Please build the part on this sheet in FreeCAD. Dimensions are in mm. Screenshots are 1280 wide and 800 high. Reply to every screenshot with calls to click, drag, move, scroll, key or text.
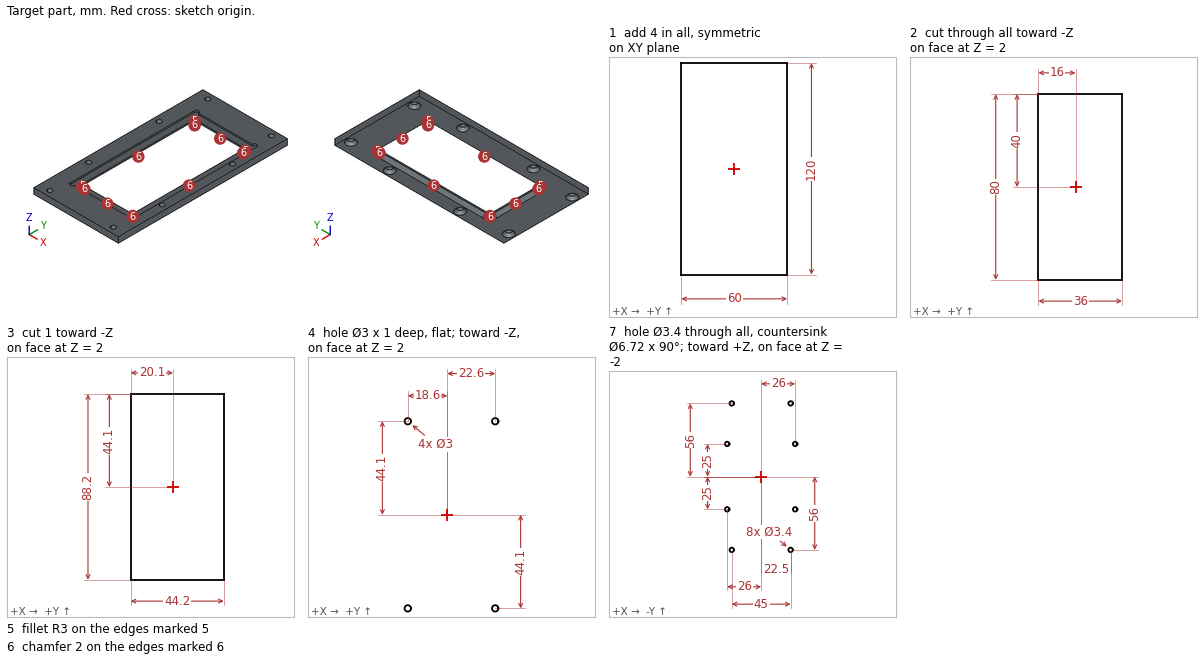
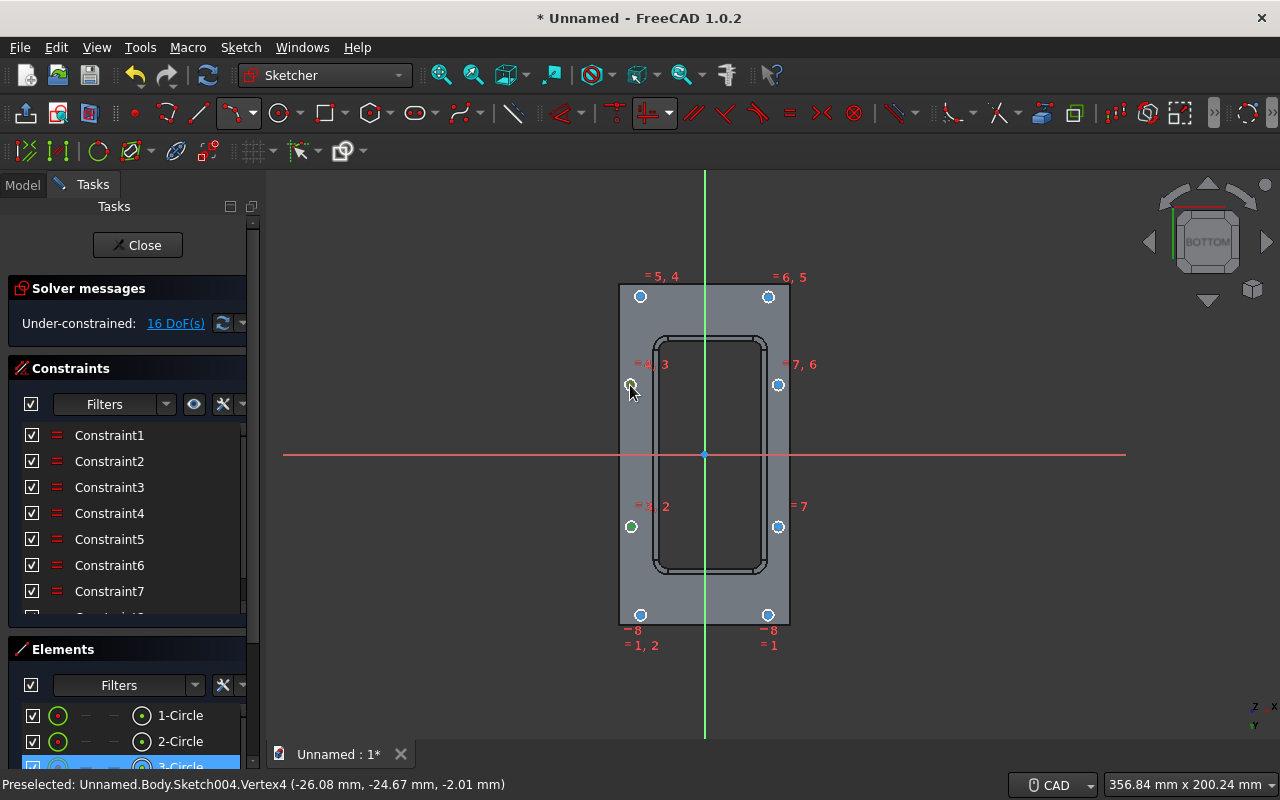
key(v)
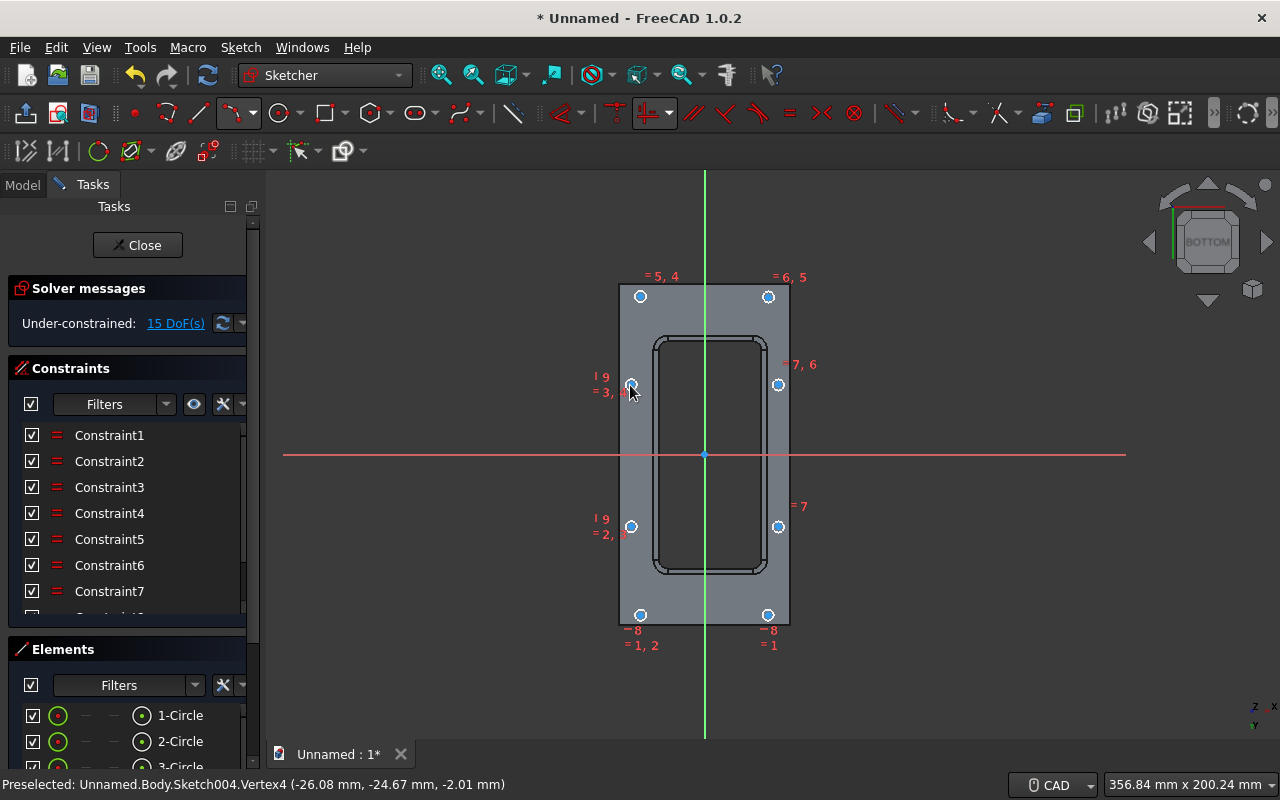
click(641, 615)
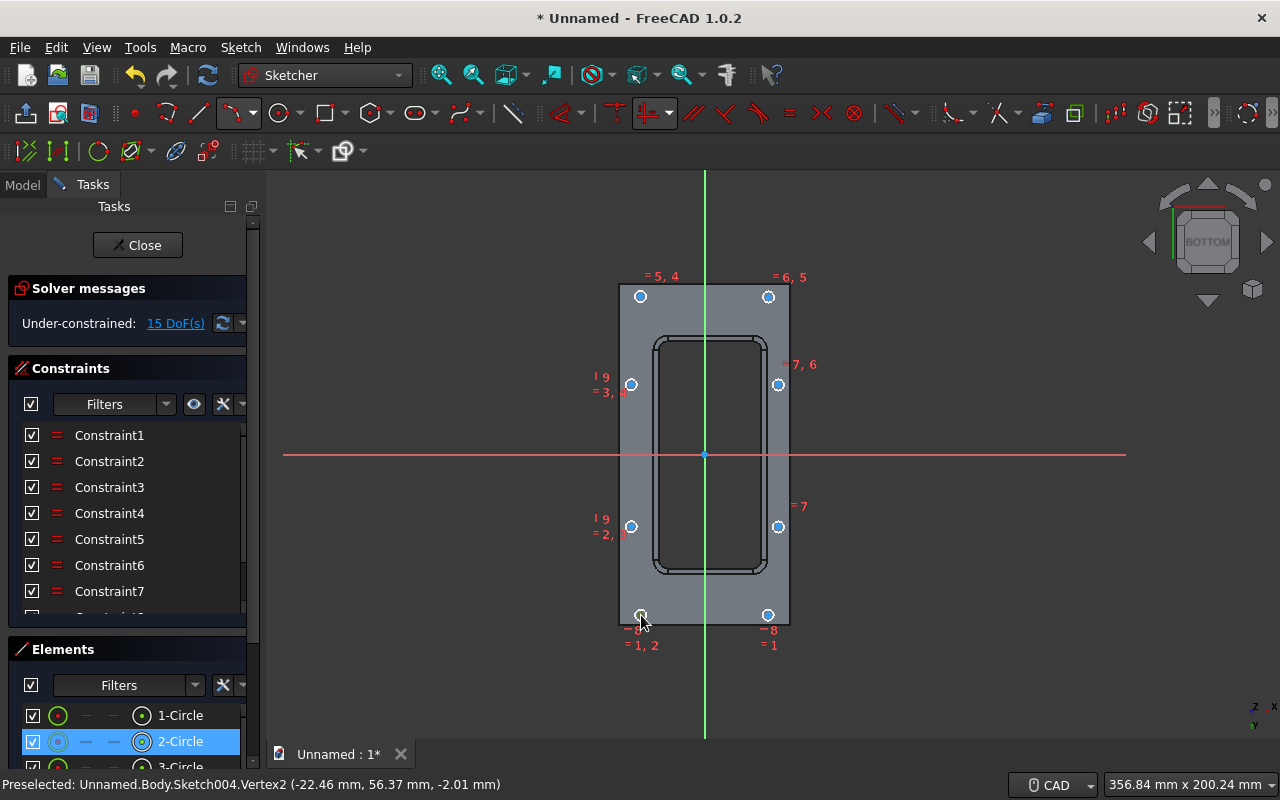
click(640, 297)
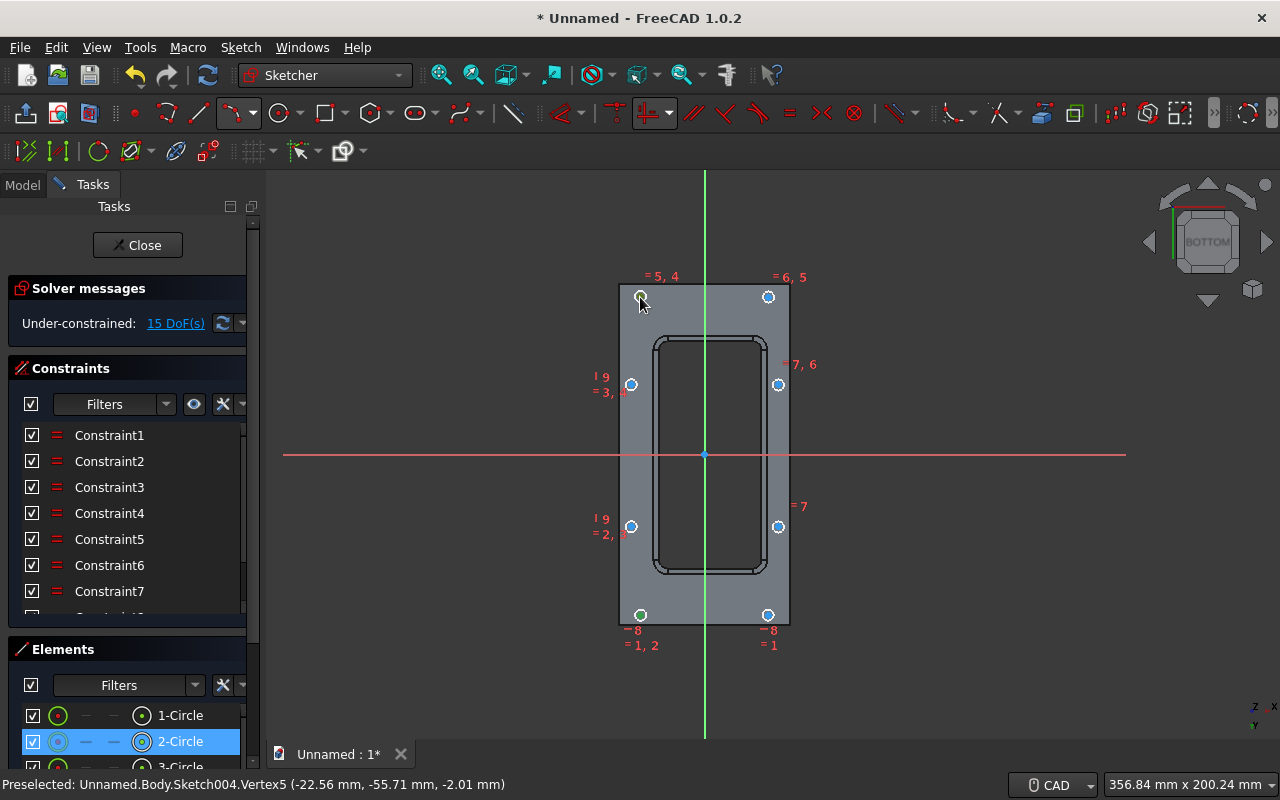
click(672, 114)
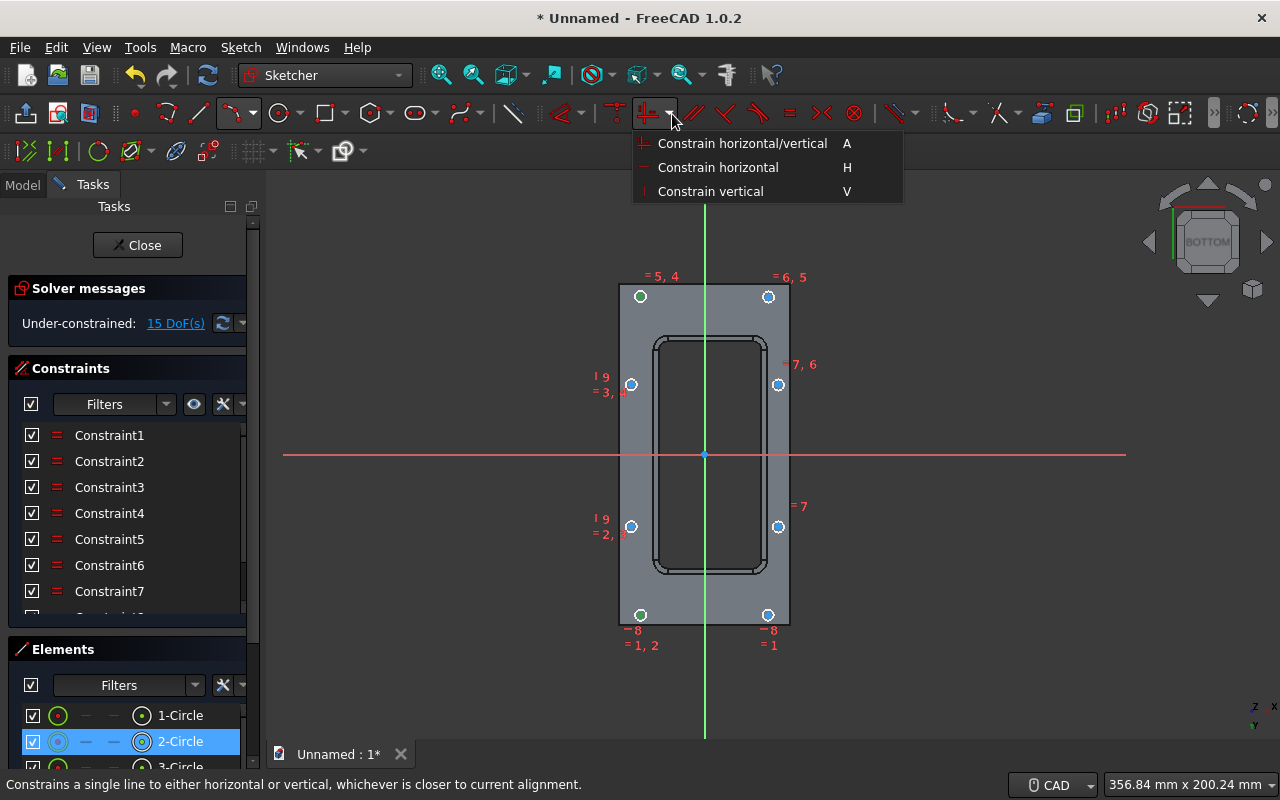
click(768, 191)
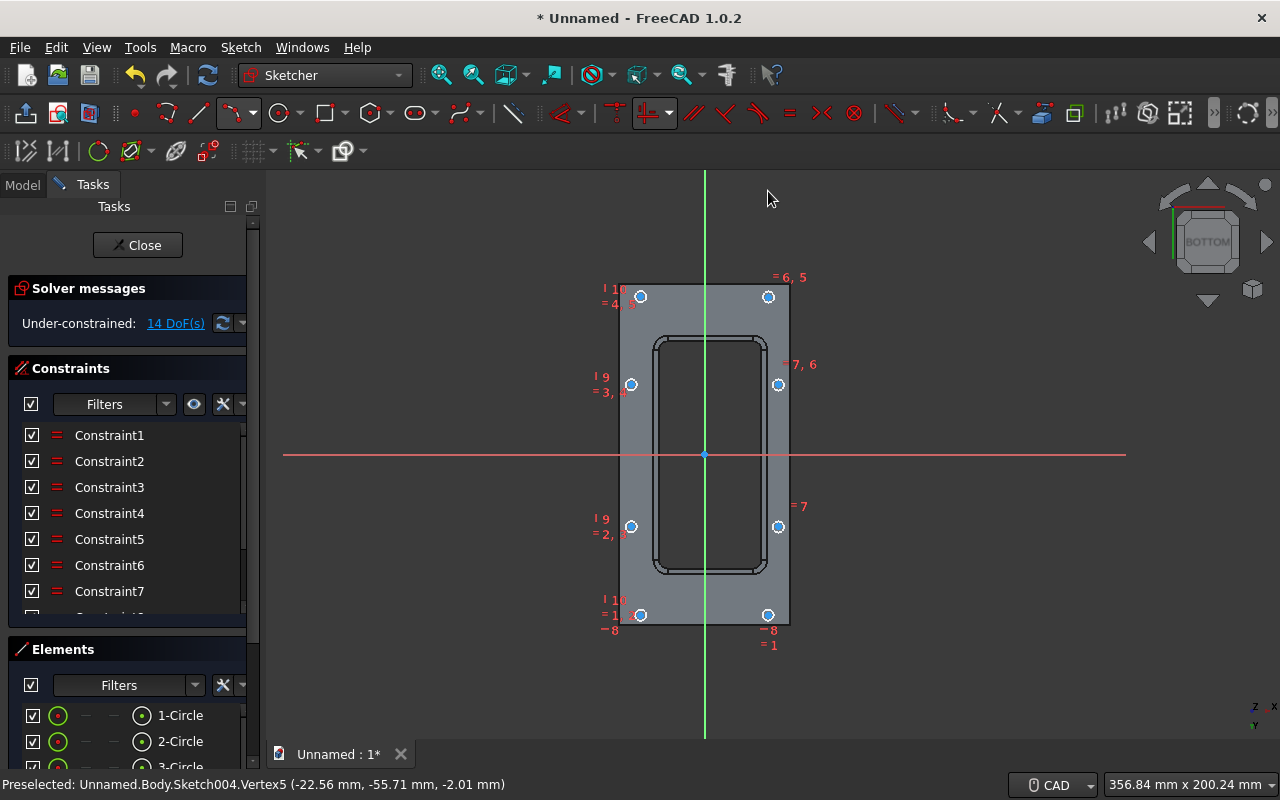
click(768, 615)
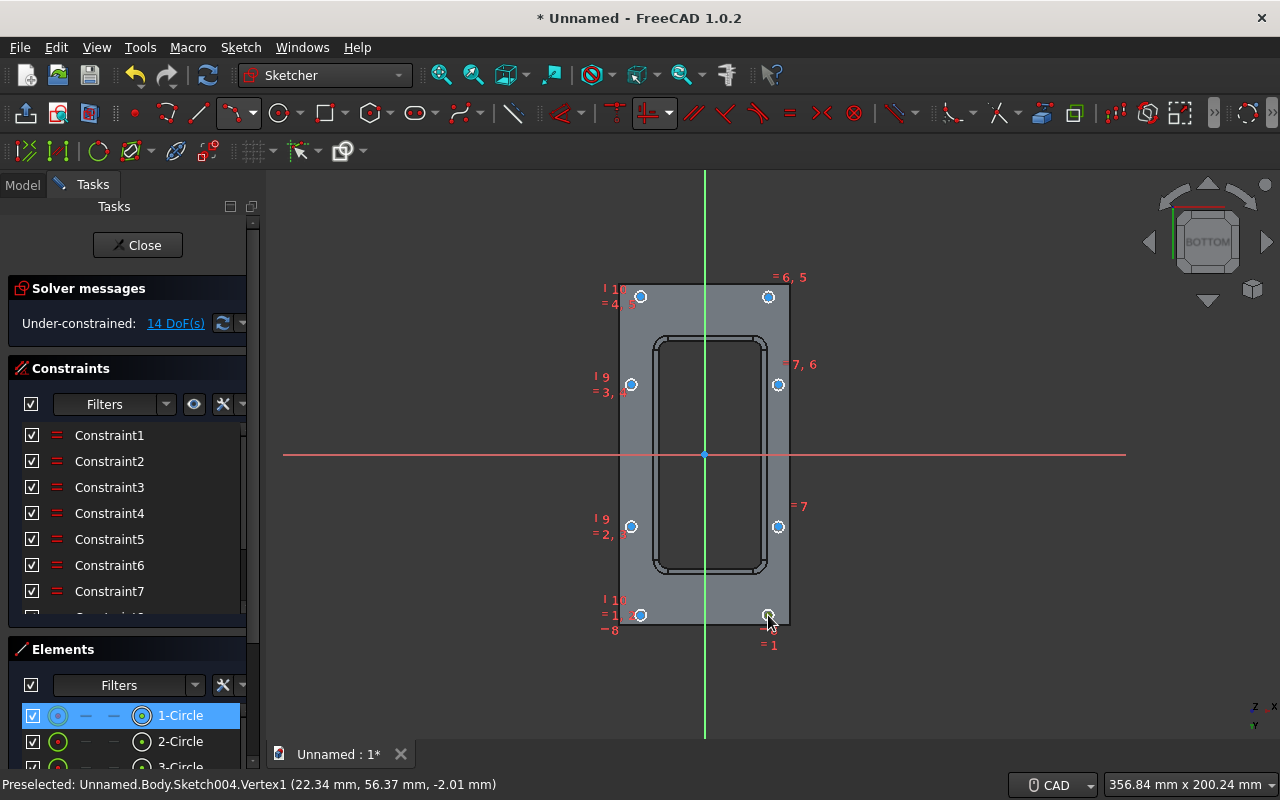
click(769, 297)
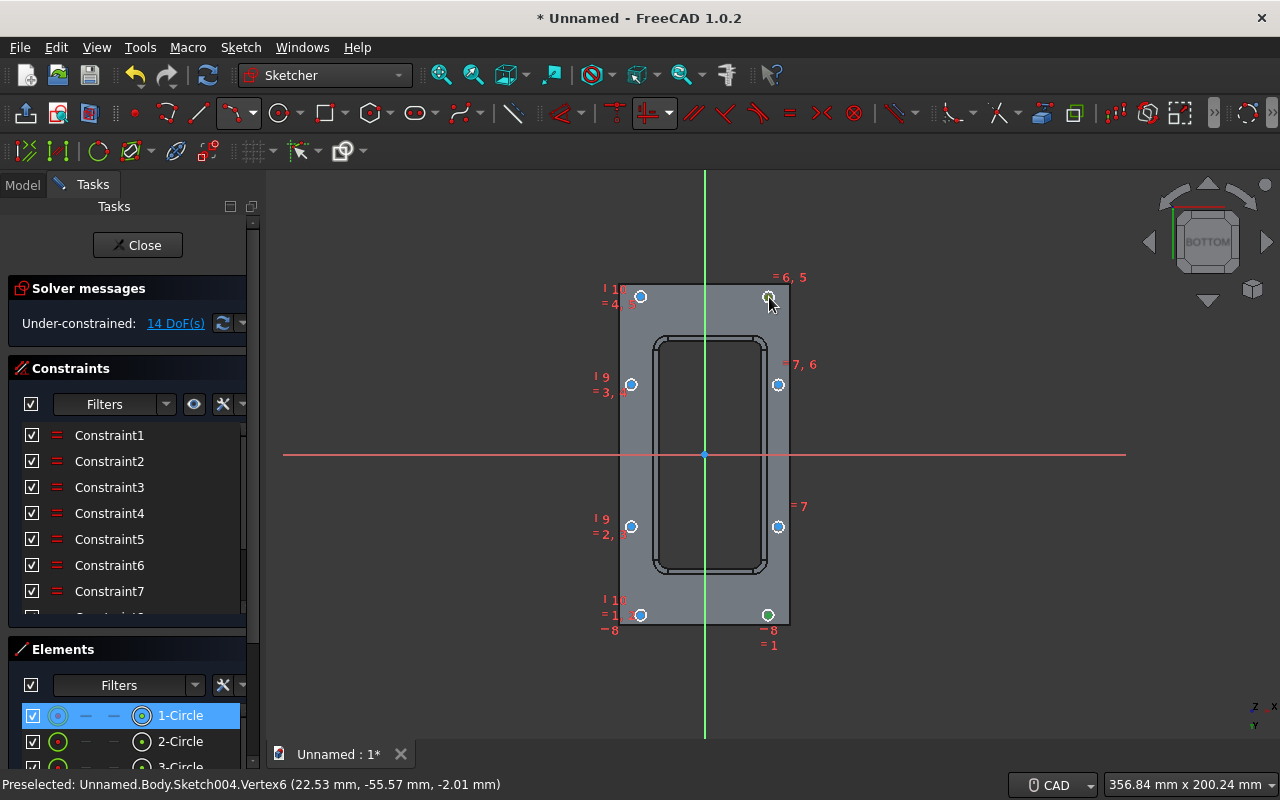
click(672, 114)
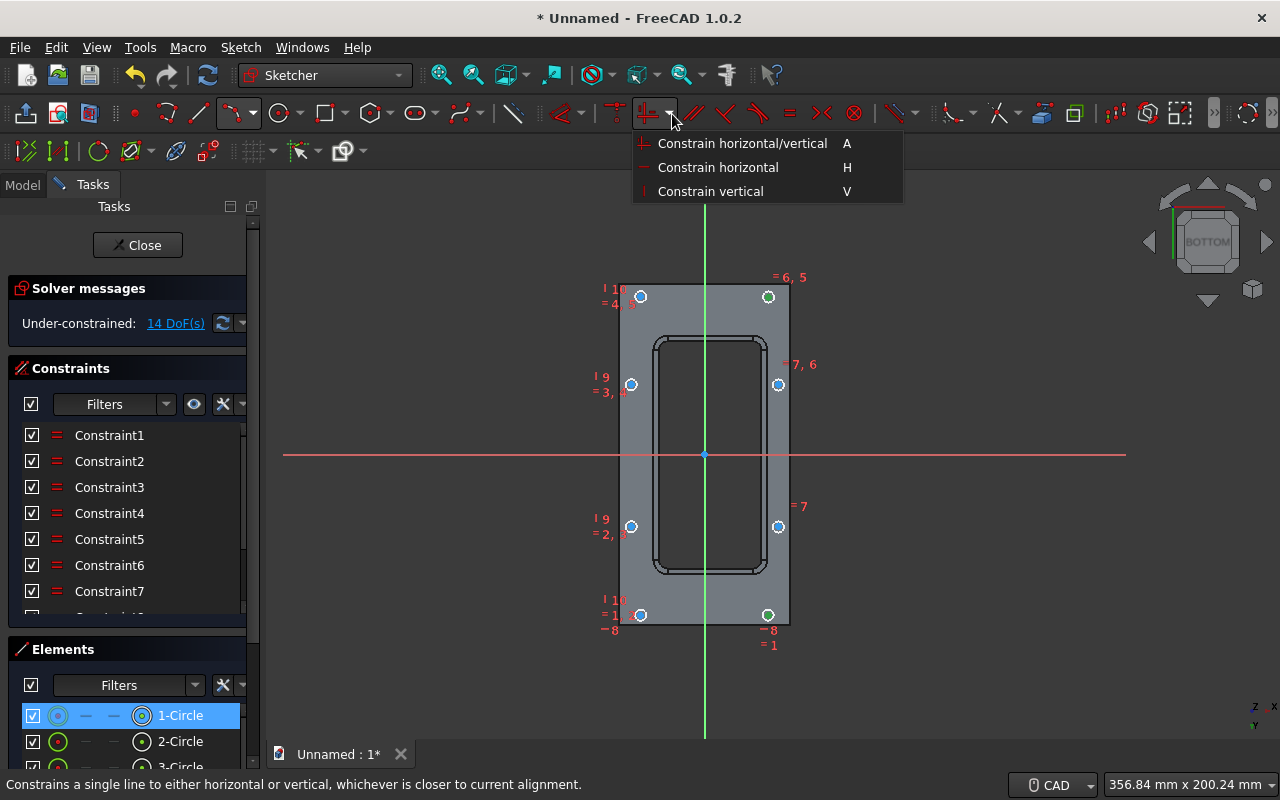
click(768, 191)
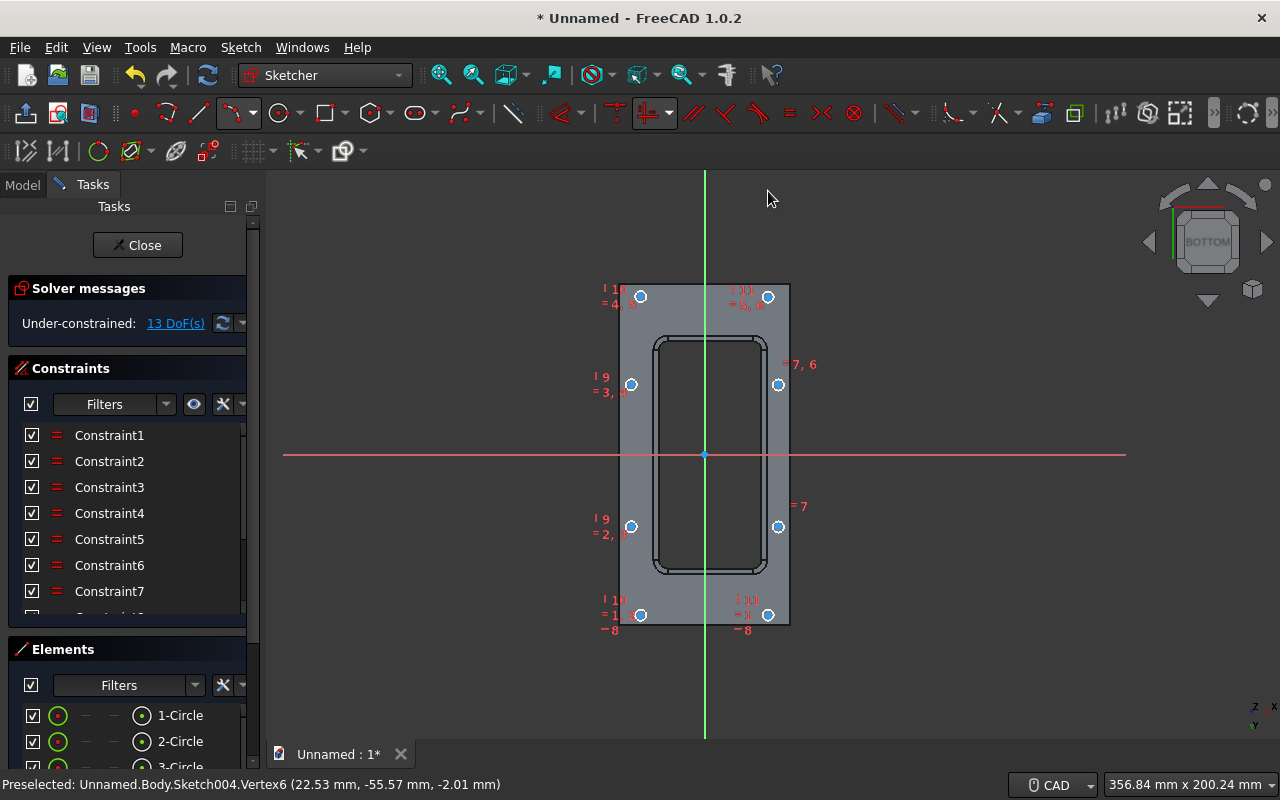
click(641, 297)